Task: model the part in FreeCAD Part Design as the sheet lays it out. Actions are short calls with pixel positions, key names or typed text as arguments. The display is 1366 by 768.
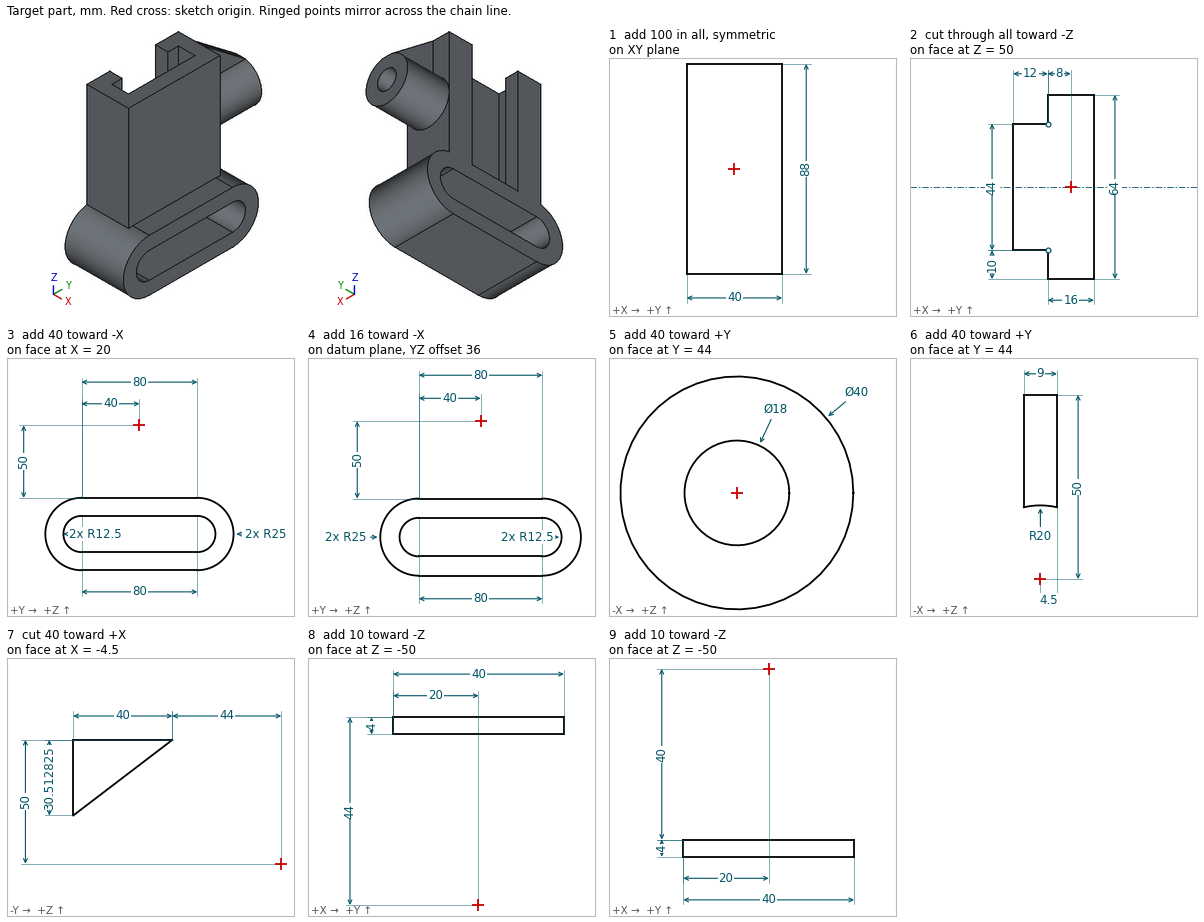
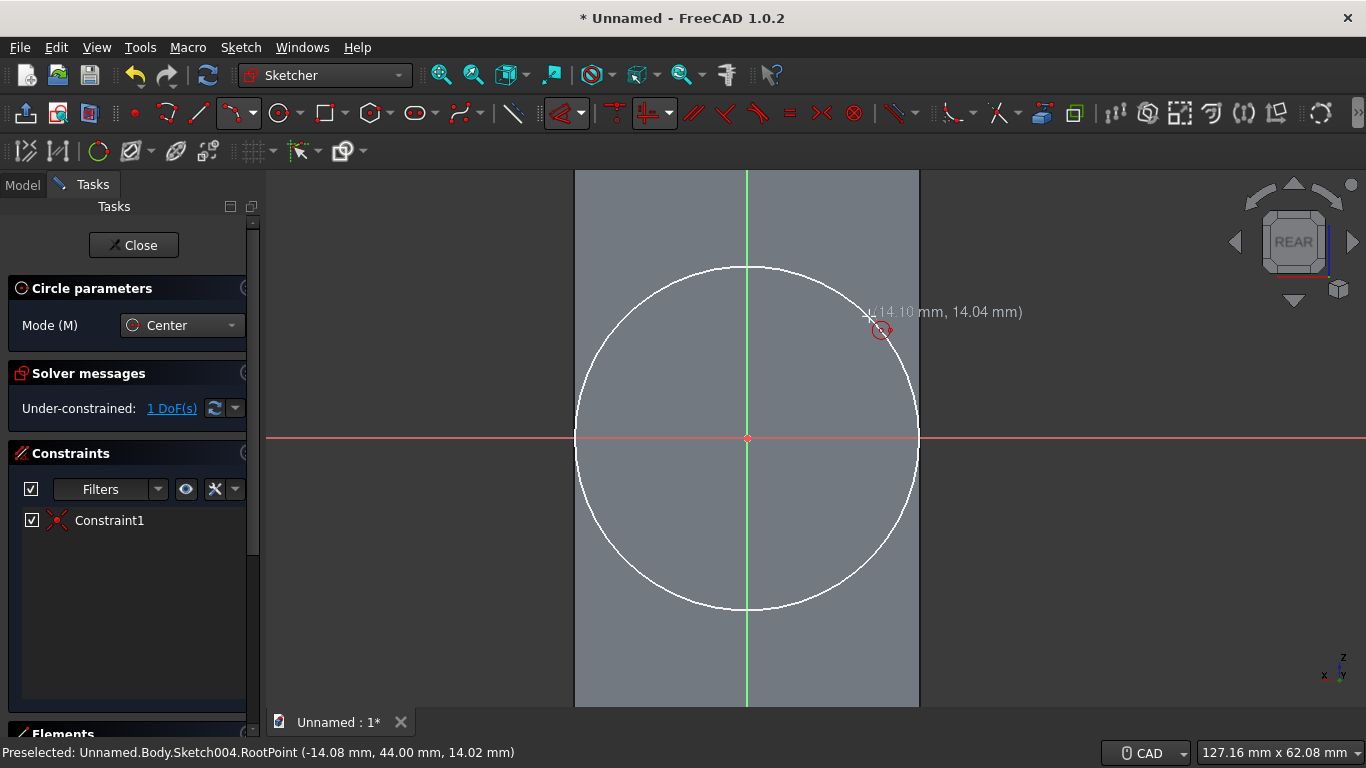
click(747, 438)
click(802, 383)
key(Escape)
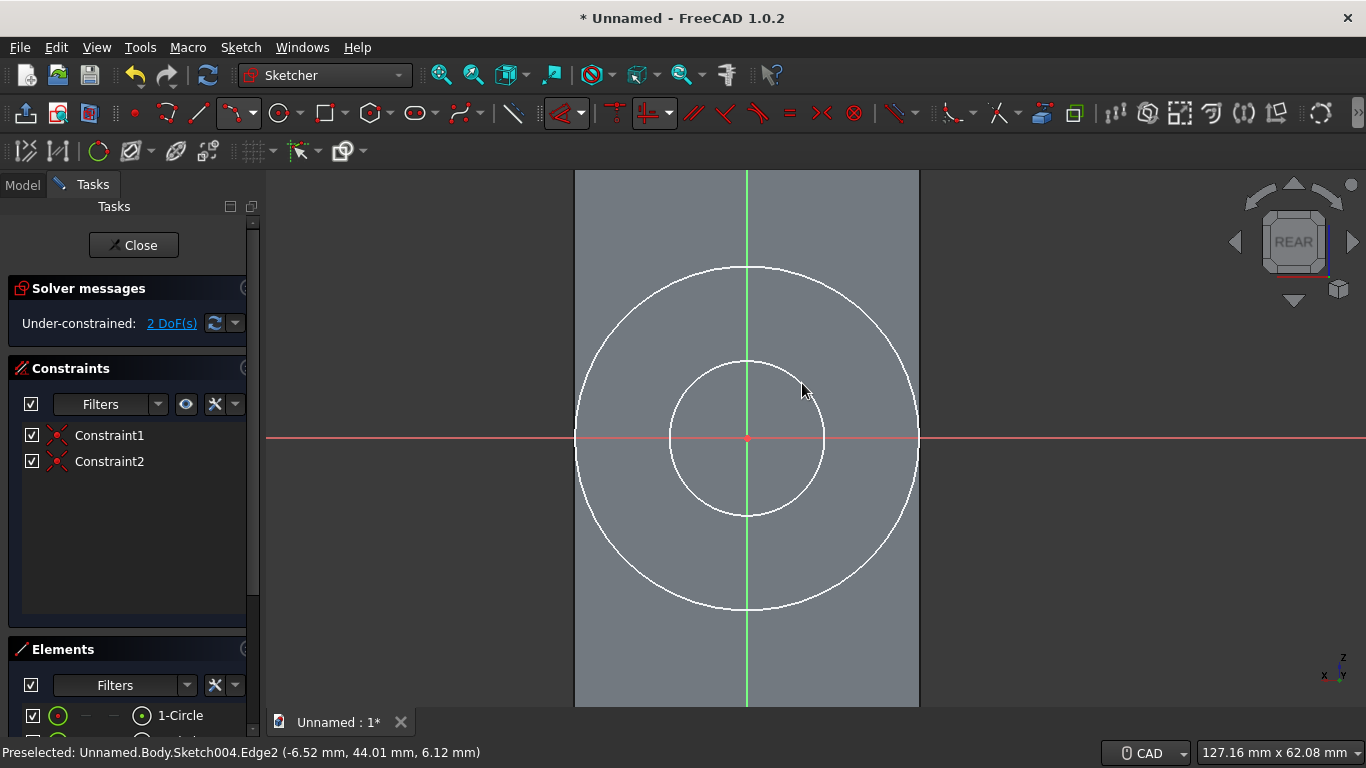
click(868, 316)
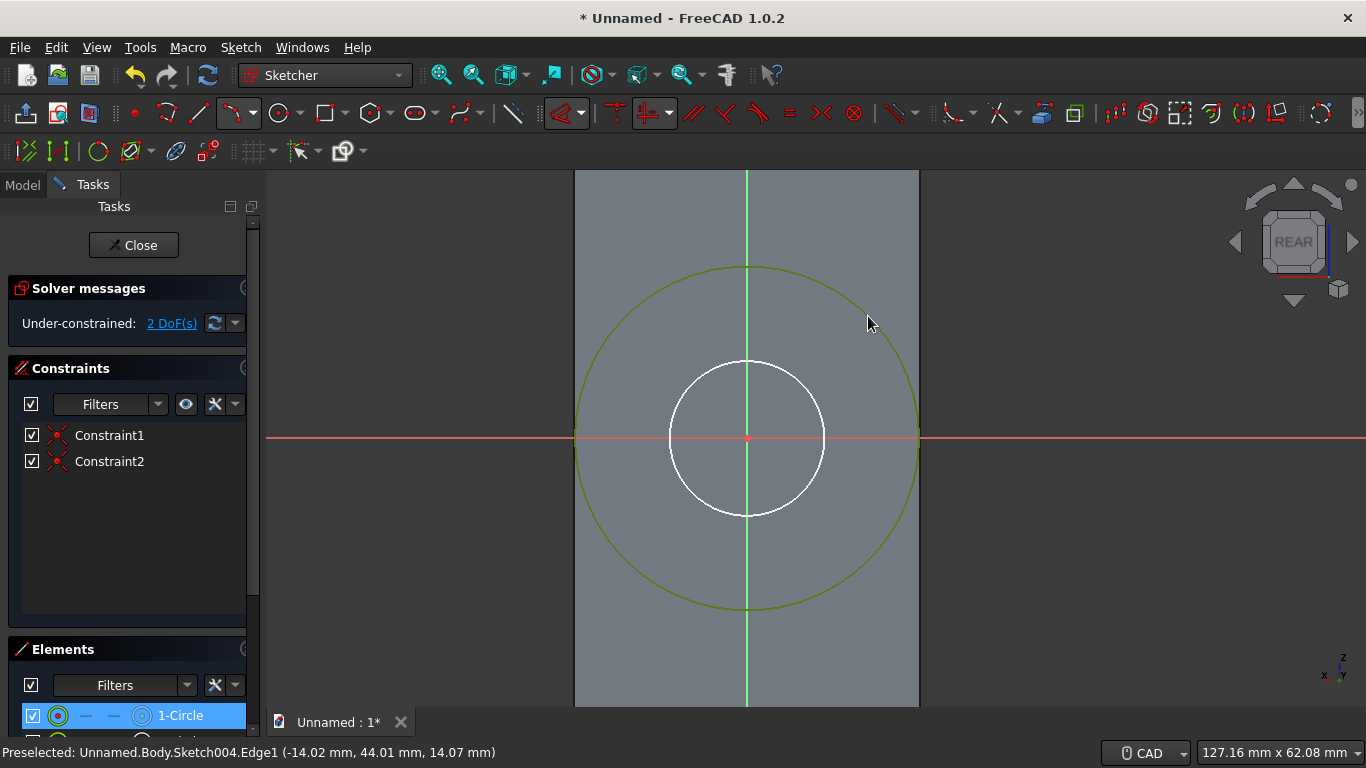
key(k)
key(o)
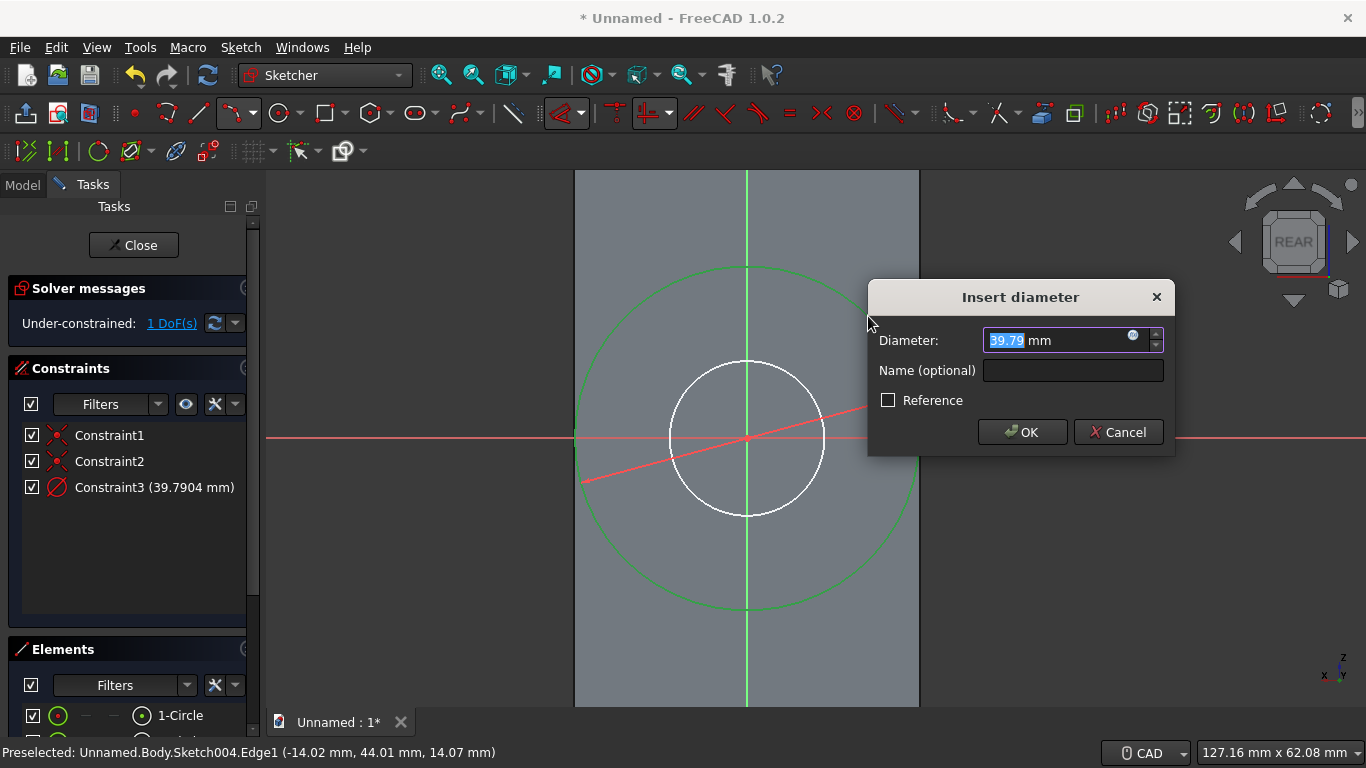
text(40)
key(Return)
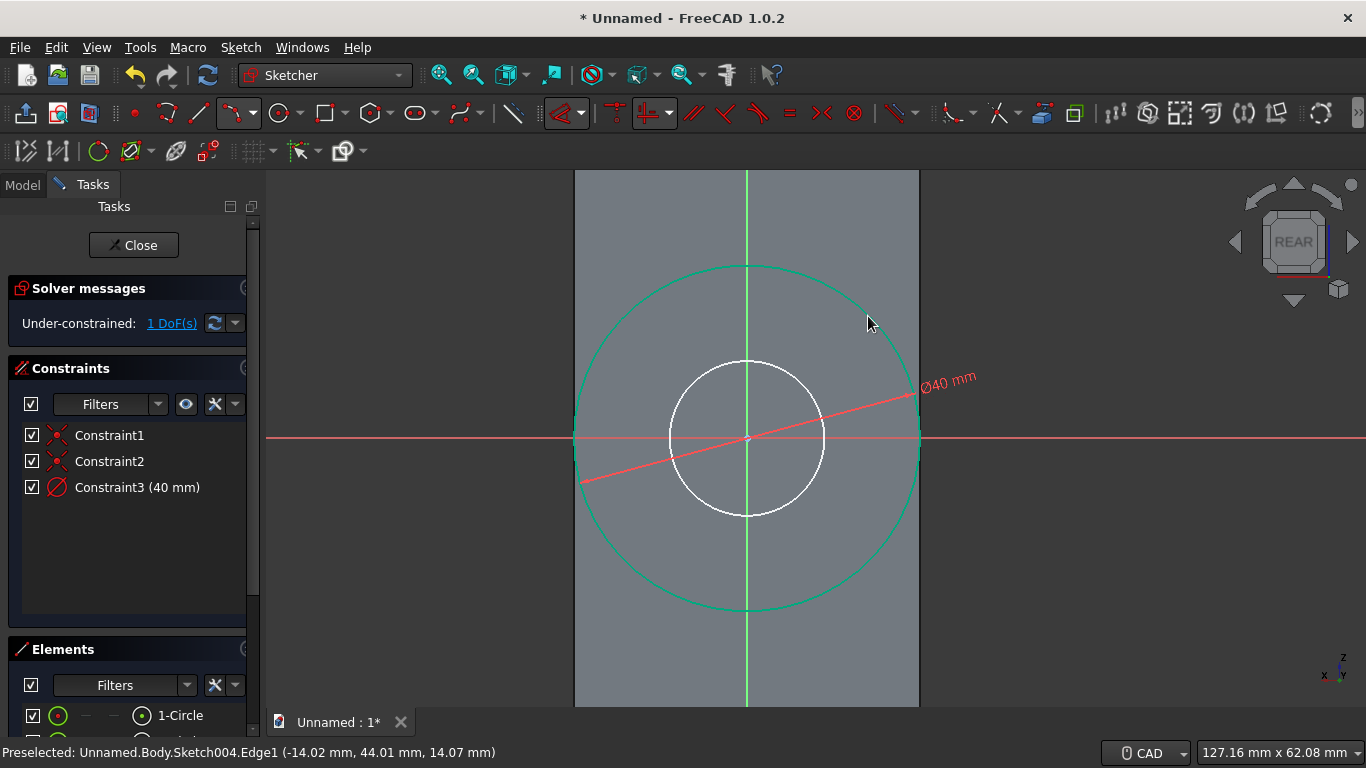
click(802, 384)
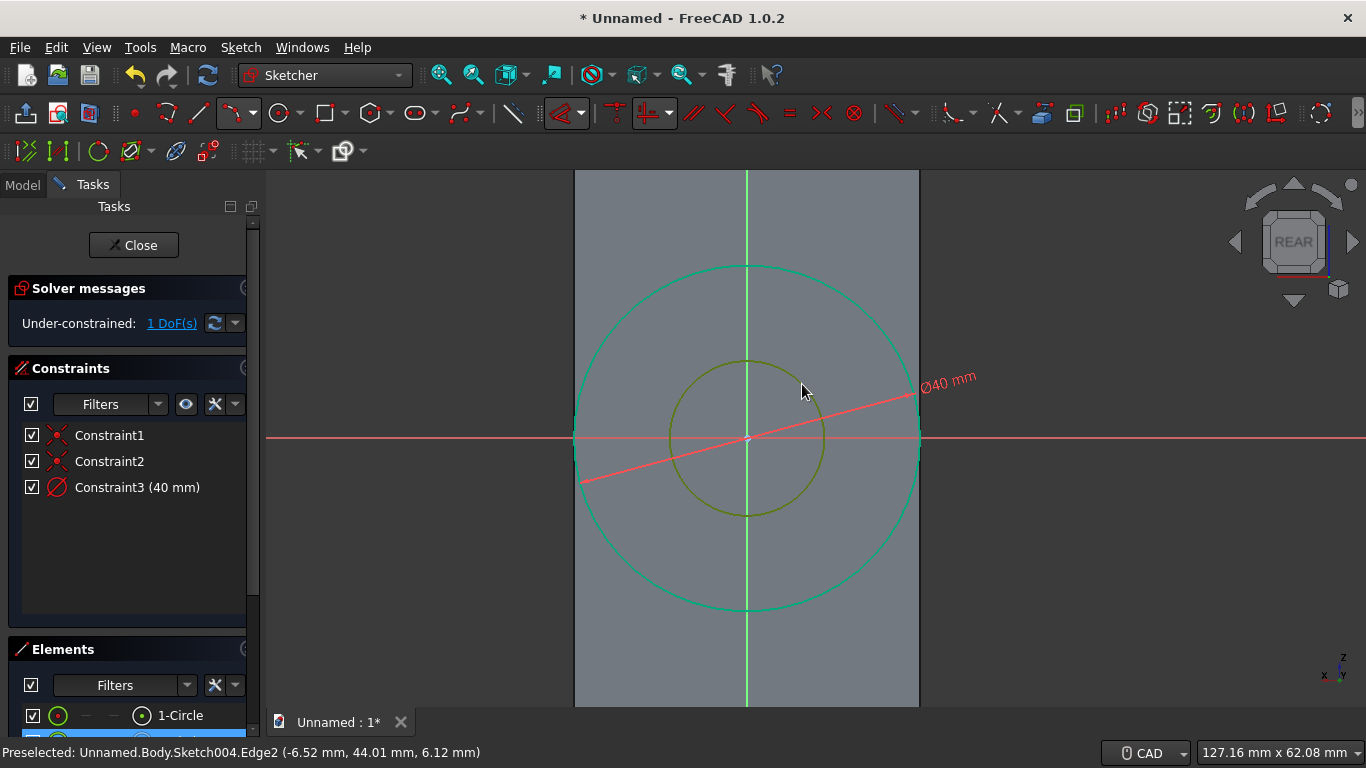
key(k)
key(o)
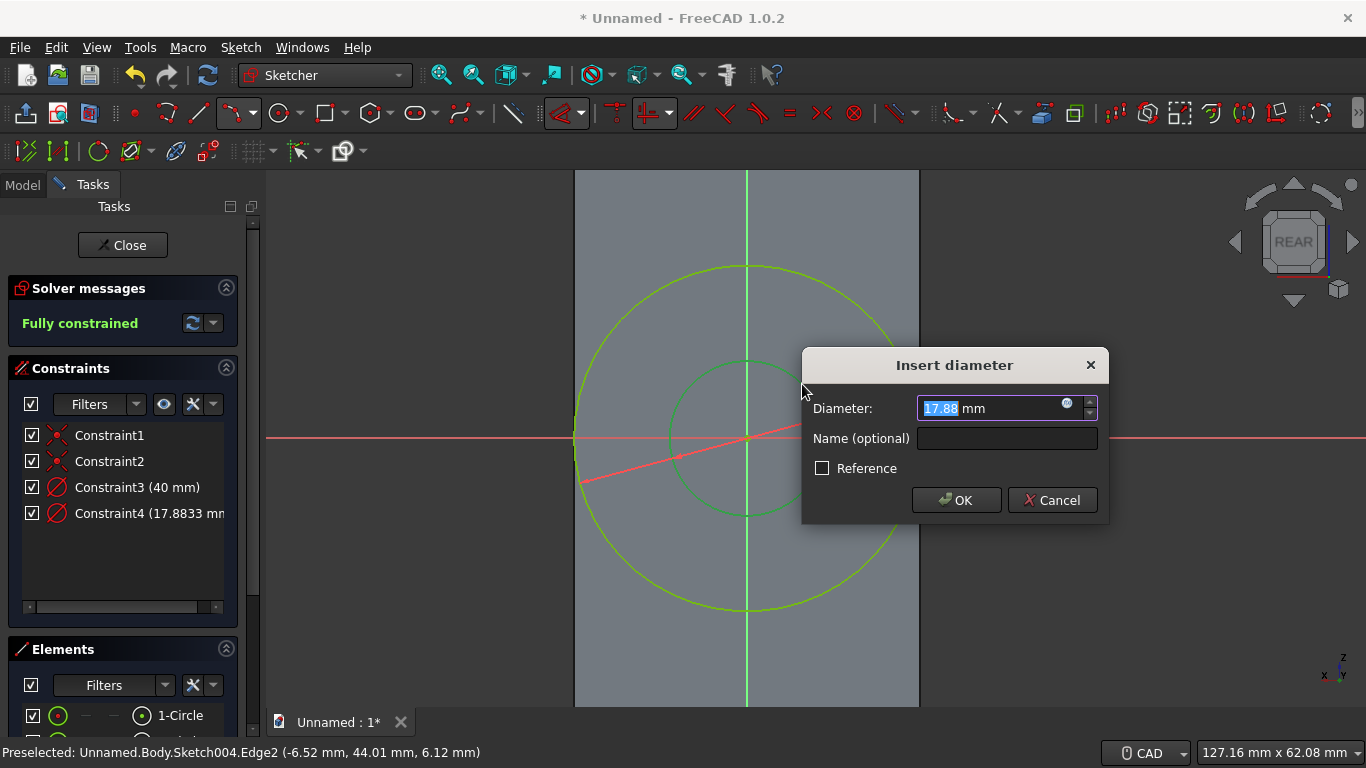
text(18)
key(Return)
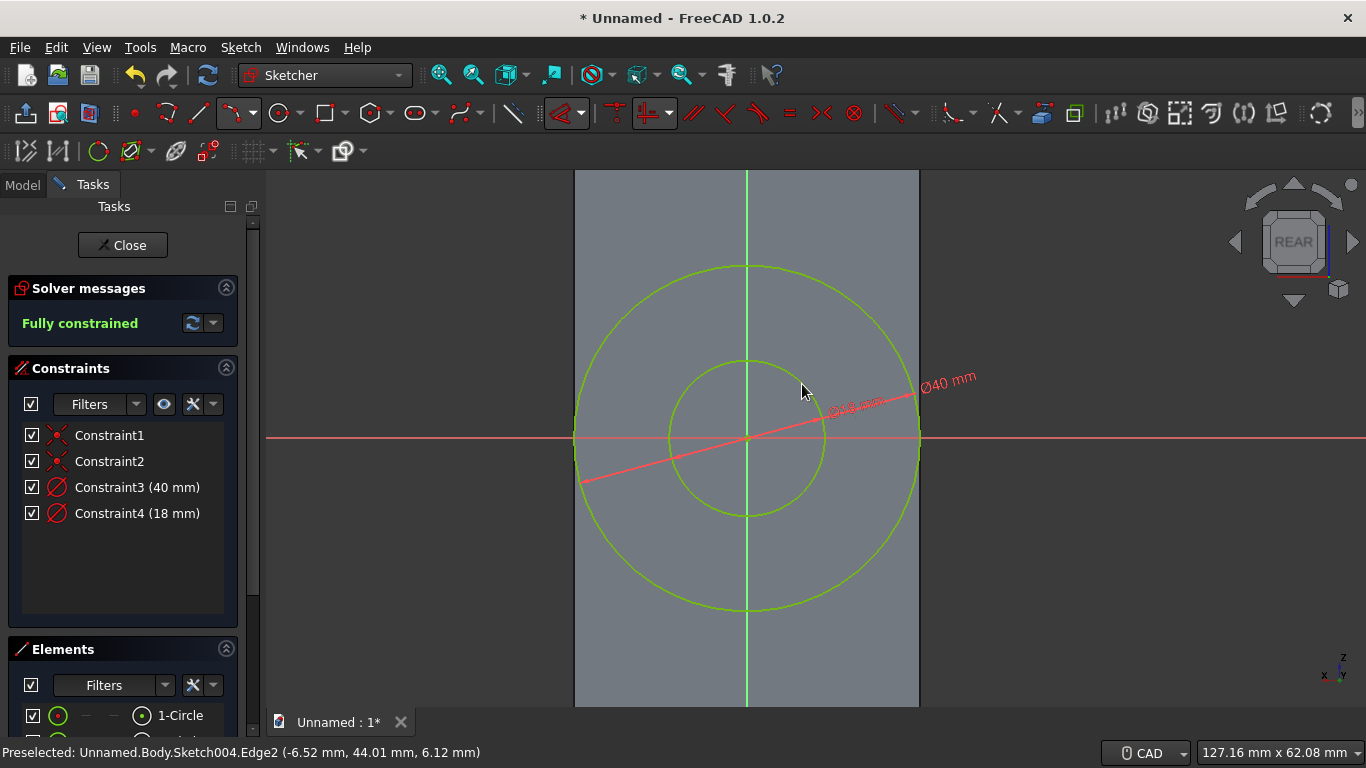
click(123, 245)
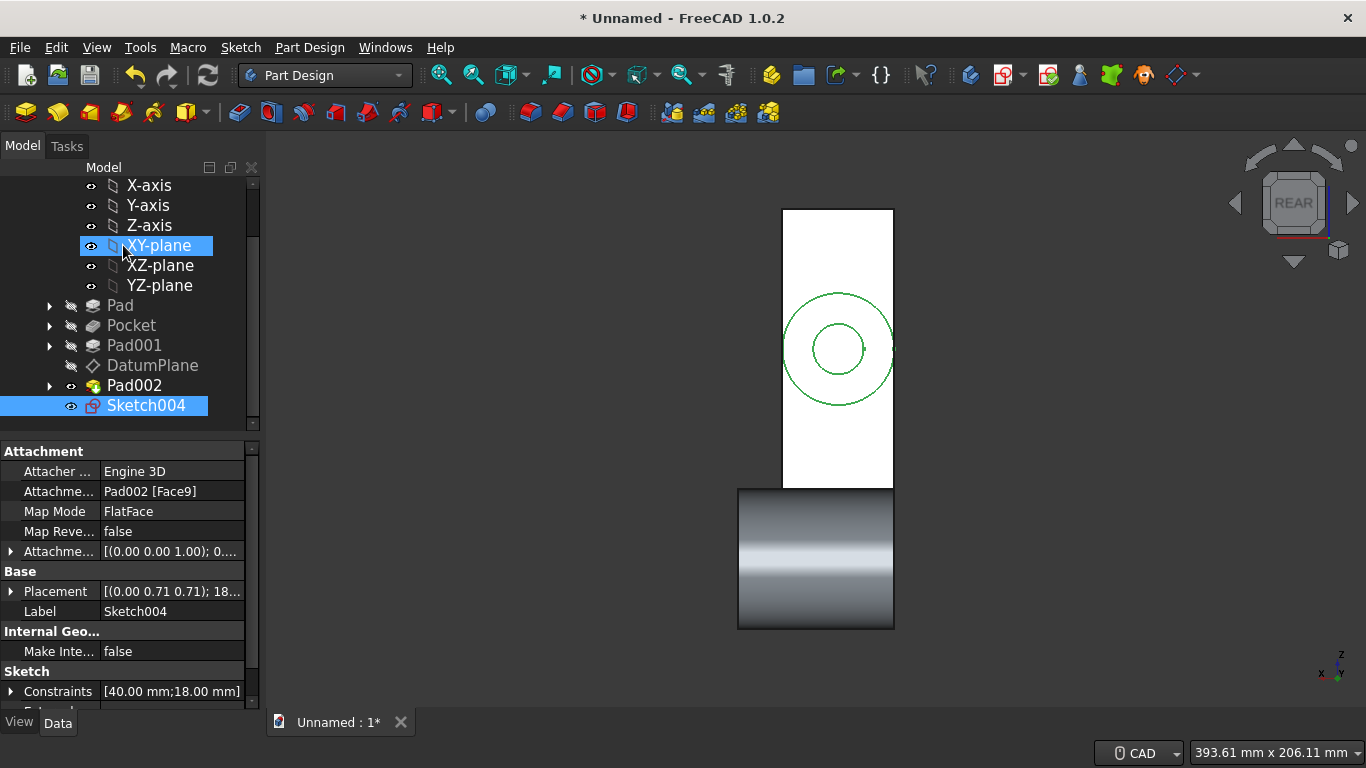
click(26, 112)